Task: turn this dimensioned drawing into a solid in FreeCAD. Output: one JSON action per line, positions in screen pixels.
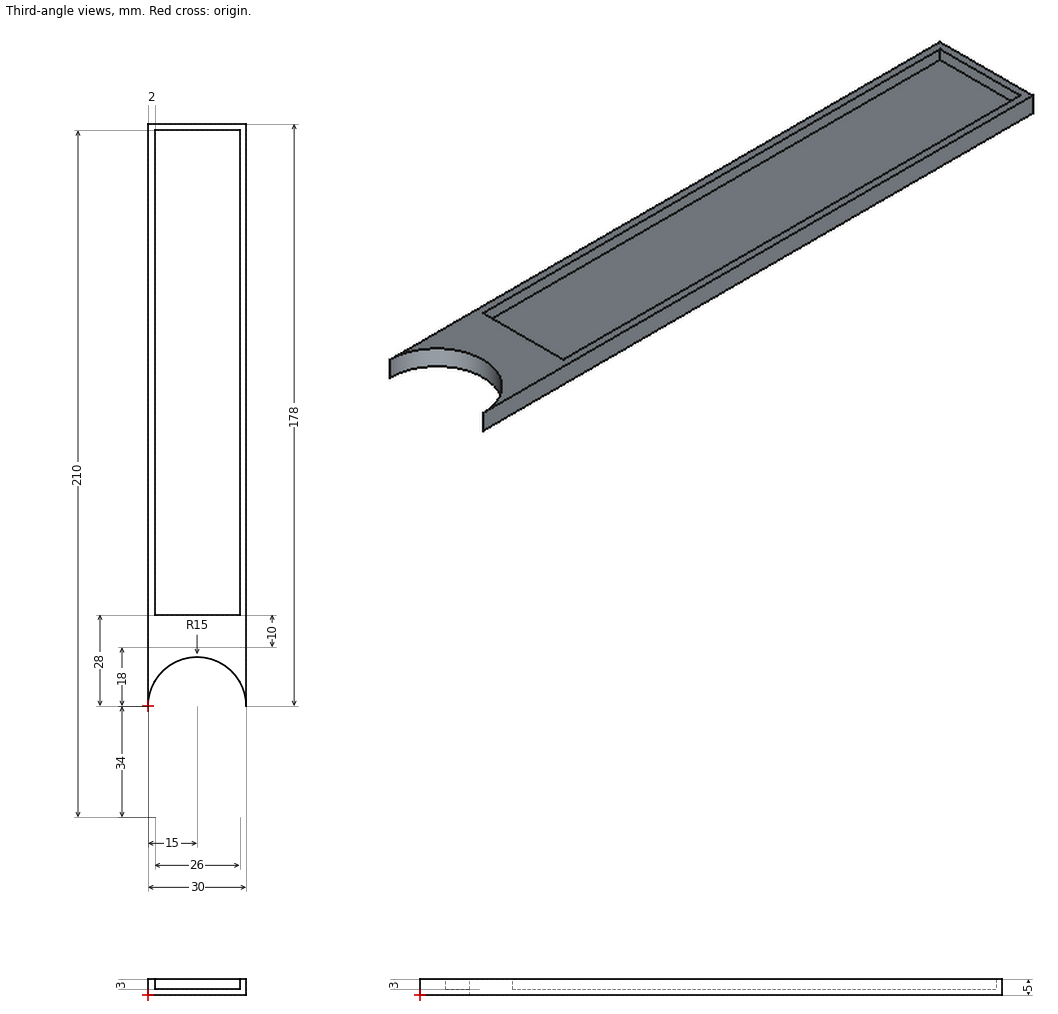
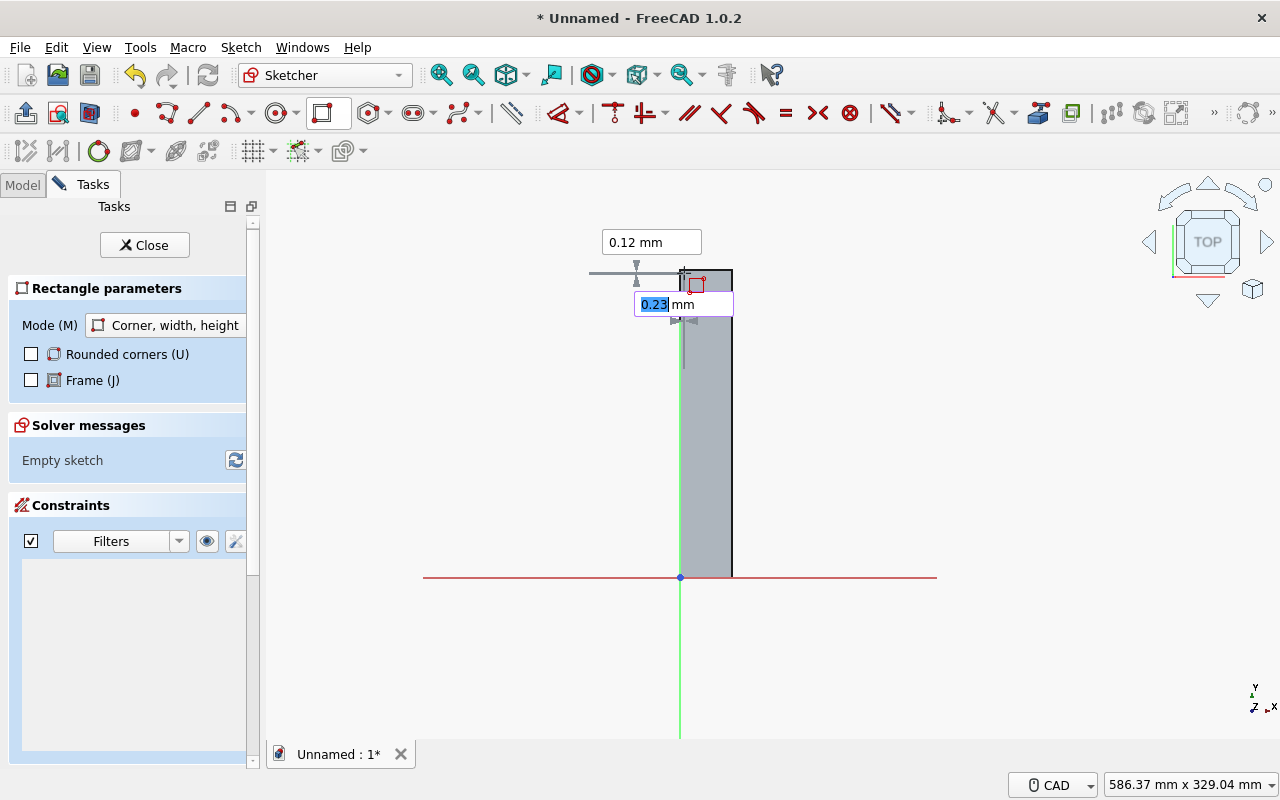
{"action": "left_click", "coordinate": [729, 636]}
{"action": "key", "text": "Escape"}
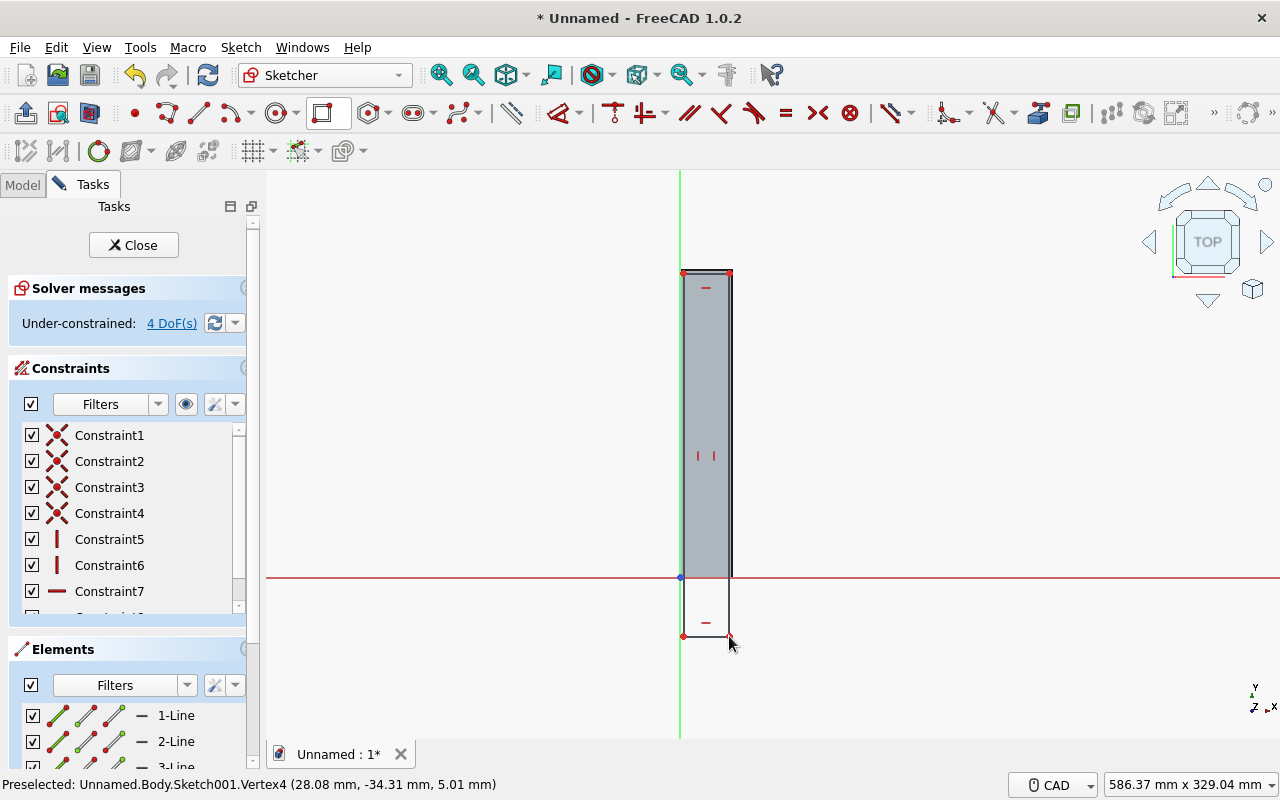
{"action": "left_click", "coordinate": [697, 637]}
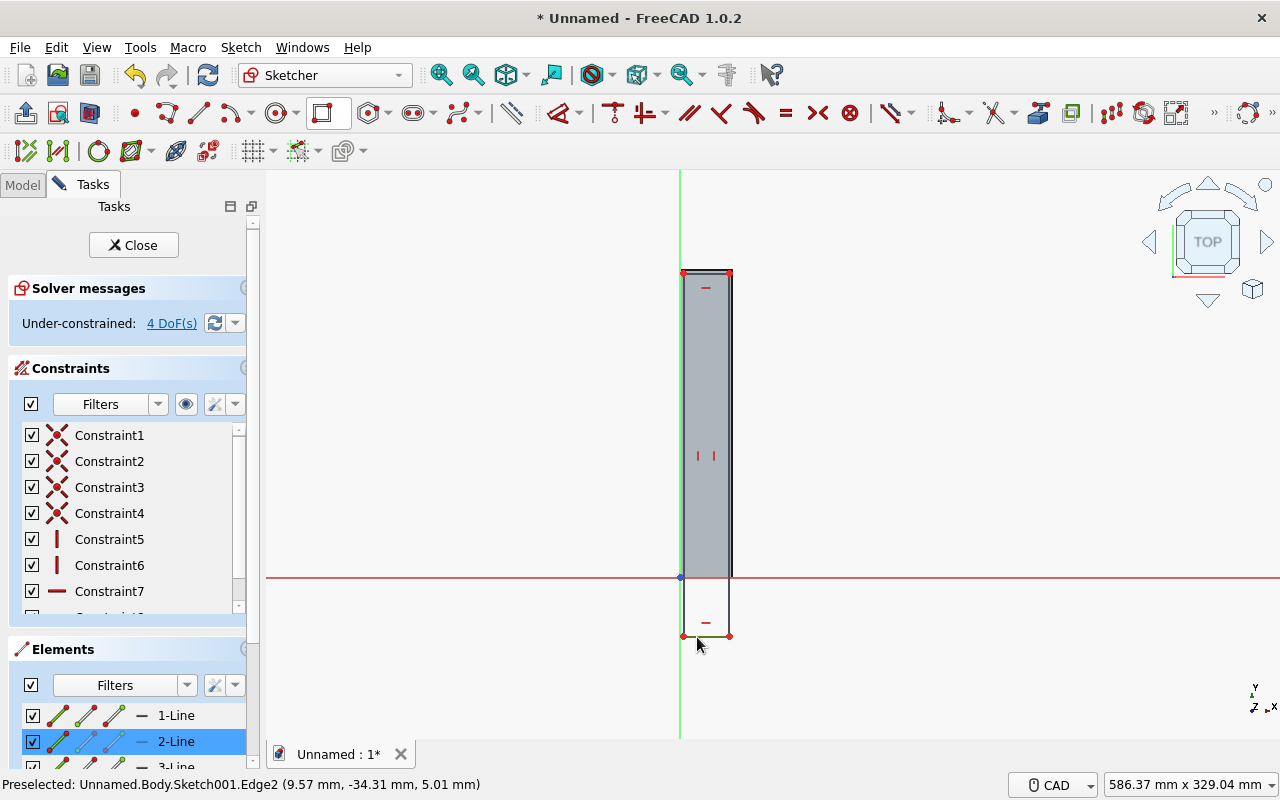
{"action": "key", "text": "l"}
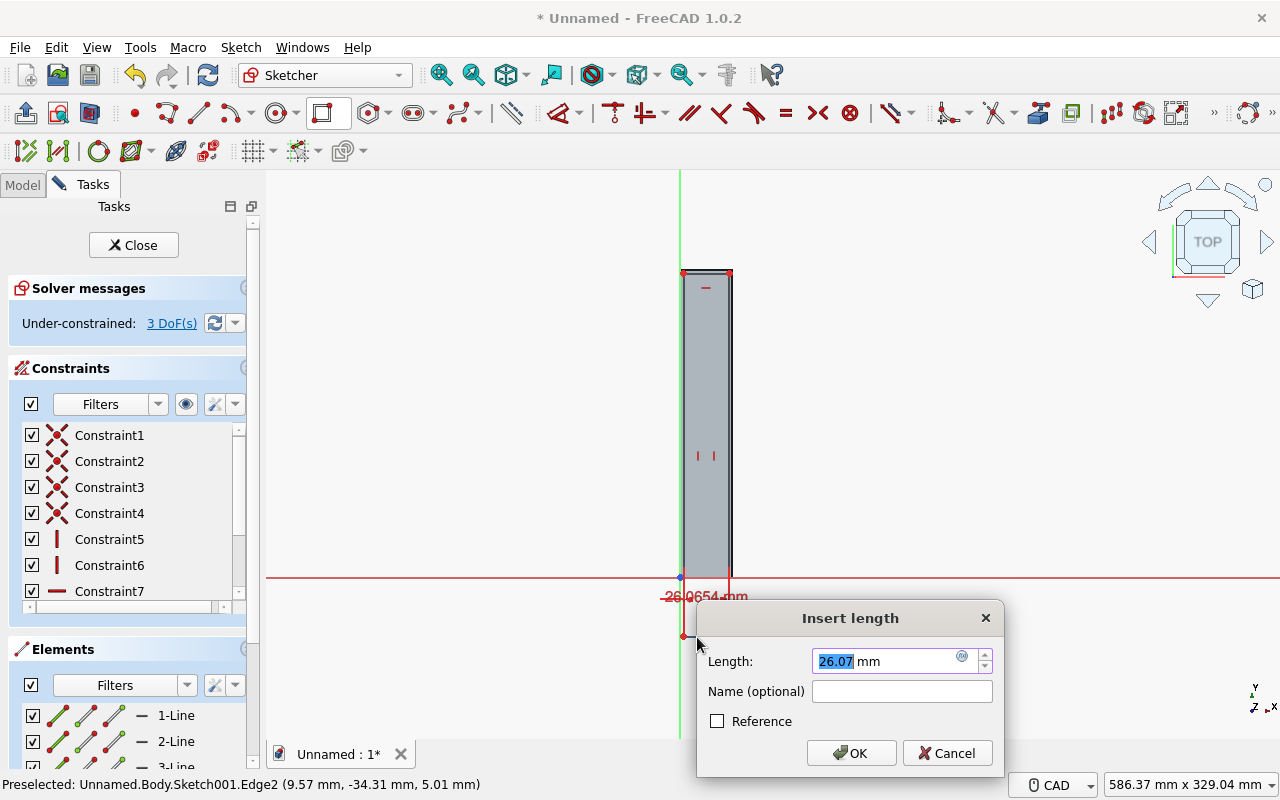
{"action": "type", "text": "26"}
{"action": "key", "text": "Return"}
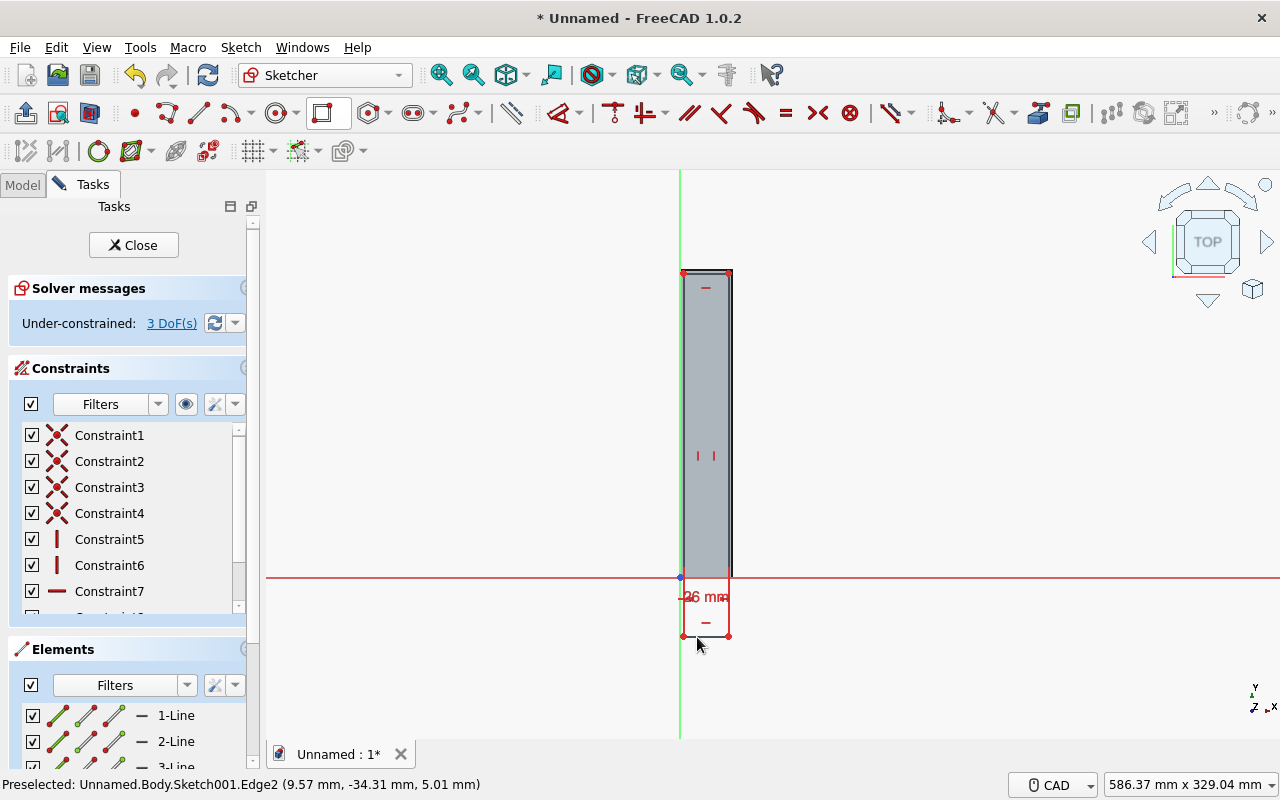
{"action": "scroll", "coordinate": [684, 274], "scroll_direction": "up", "scroll_amount": 13}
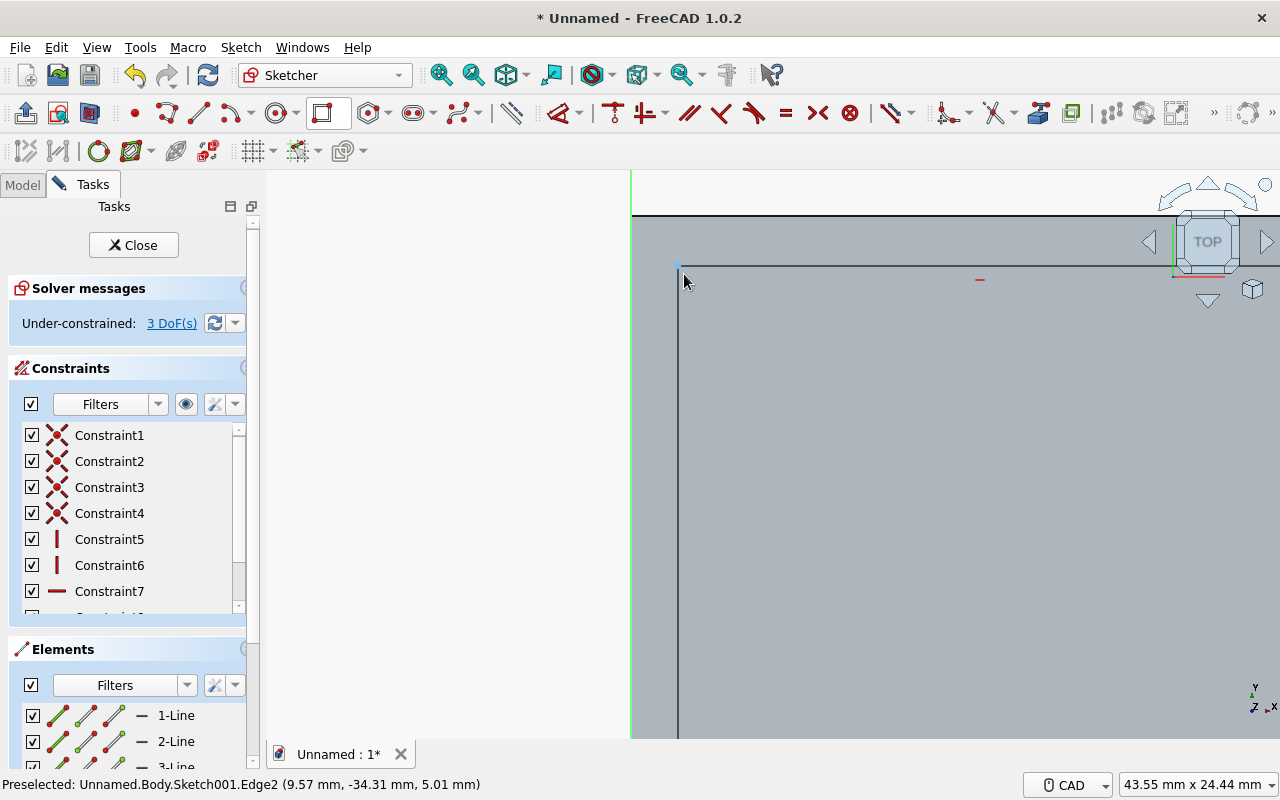
{"action": "left_click", "coordinate": [678, 266]}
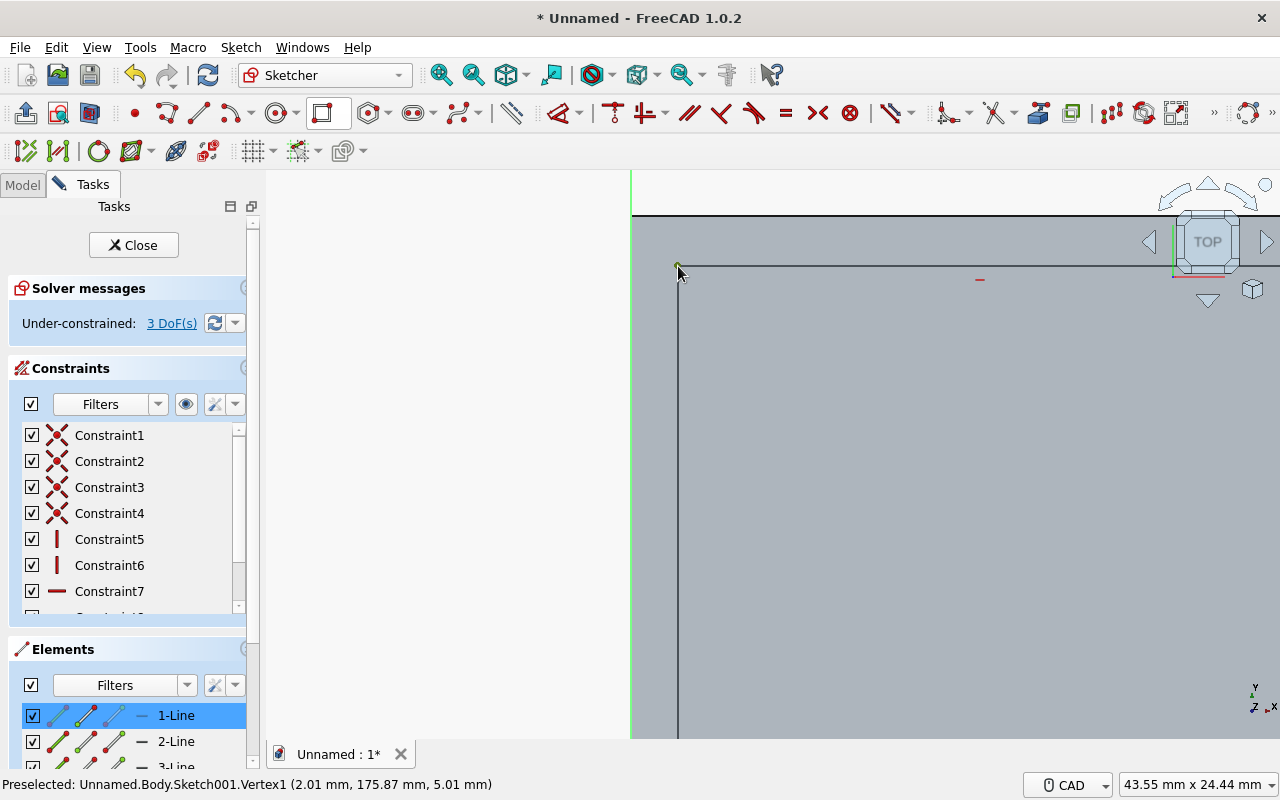
{"action": "key", "text": "l"}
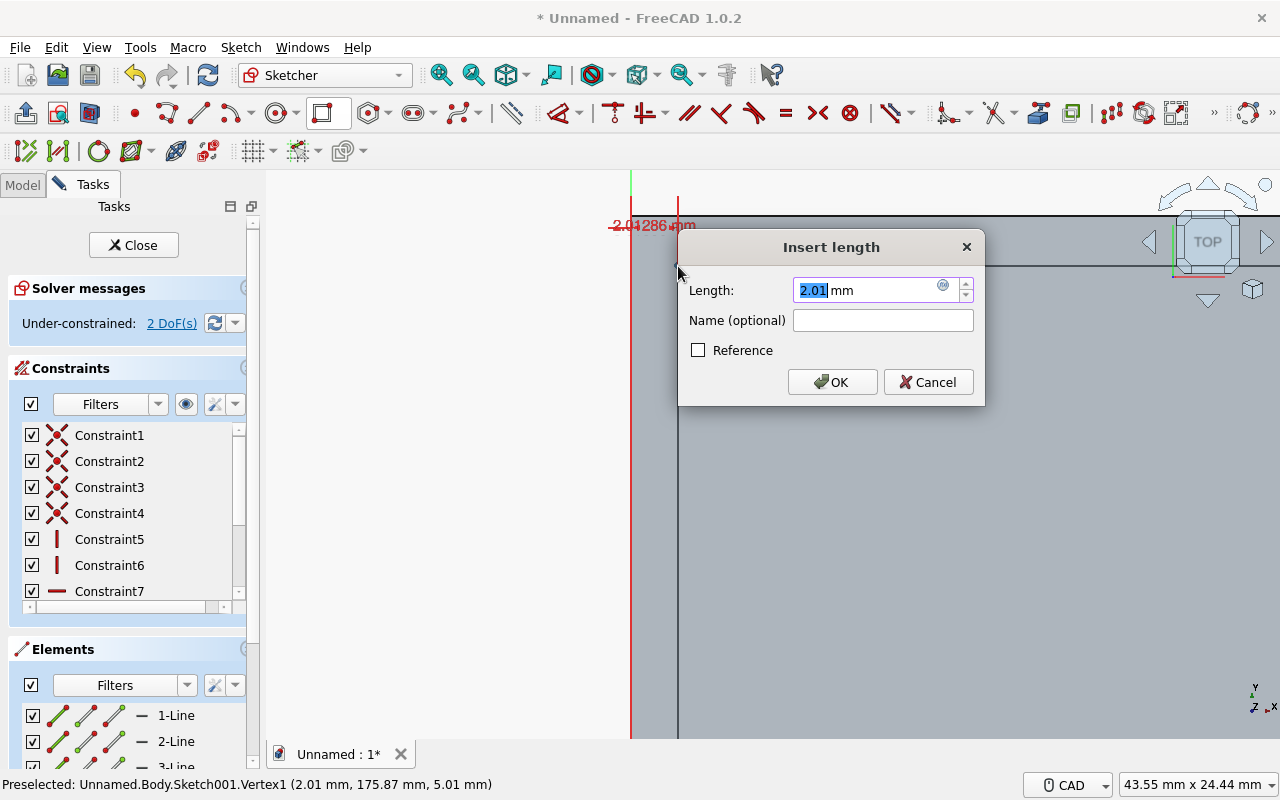
{"action": "type", "text": "2"}
{"action": "key", "text": "Return"}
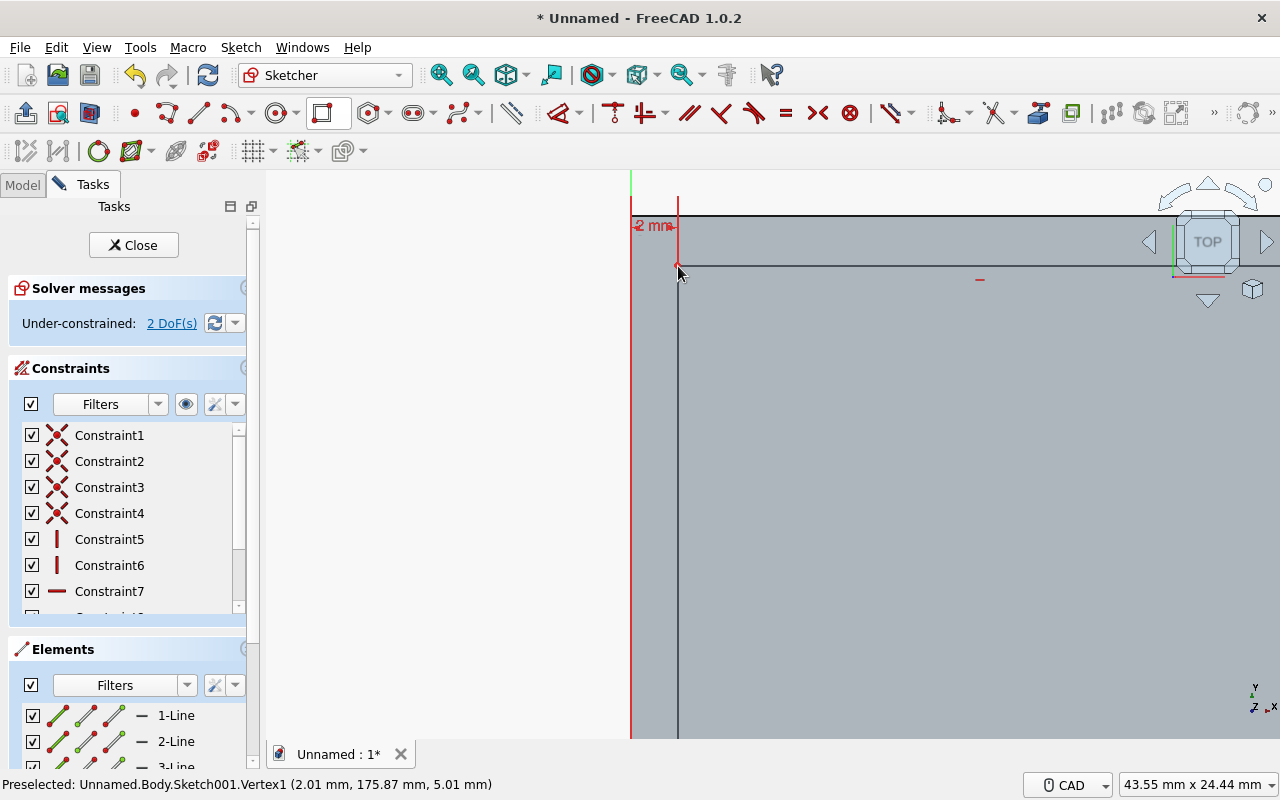
{"action": "scroll", "coordinate": [684, 274], "scroll_direction": "down", "scroll_amount": 13}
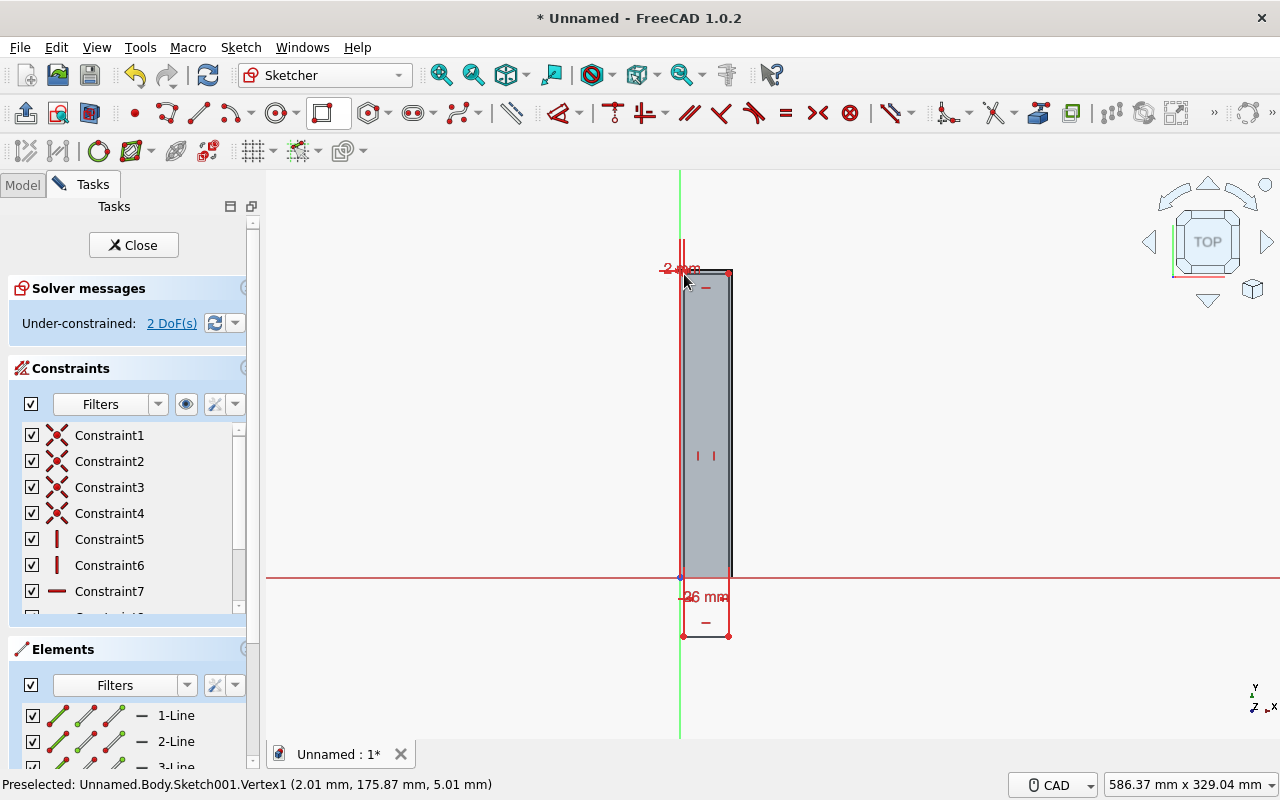
{"action": "scroll", "coordinate": [684, 383], "scroll_direction": "up", "scroll_amount": 7}